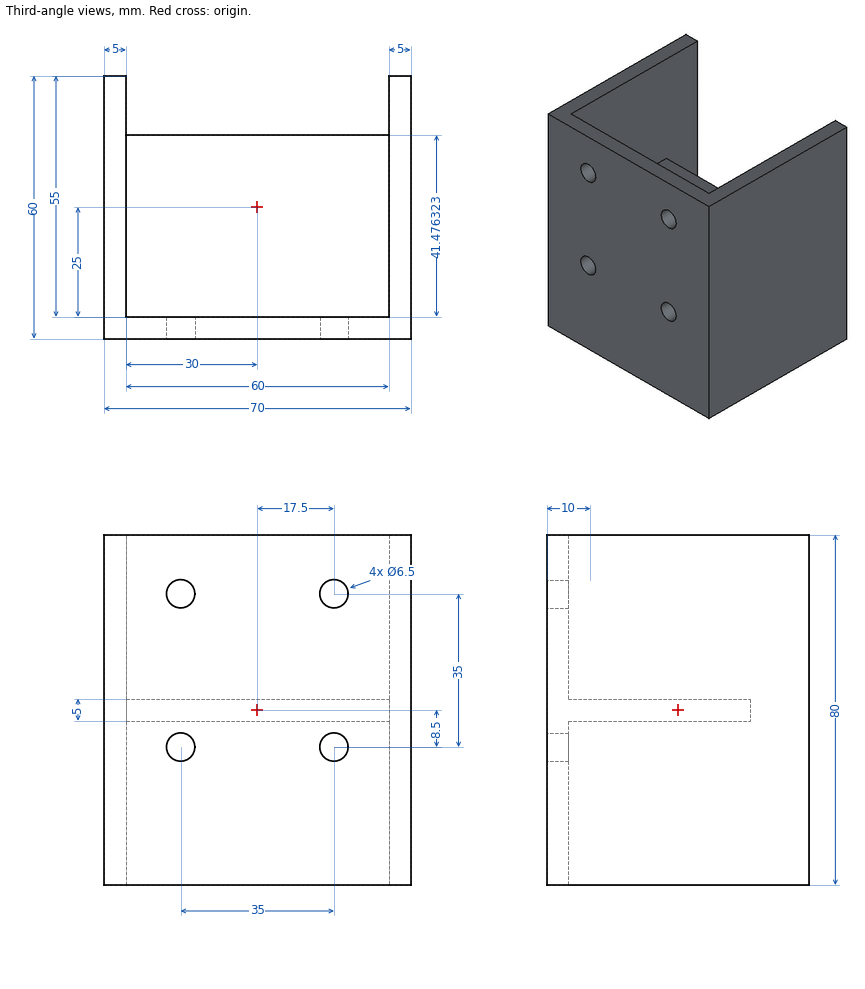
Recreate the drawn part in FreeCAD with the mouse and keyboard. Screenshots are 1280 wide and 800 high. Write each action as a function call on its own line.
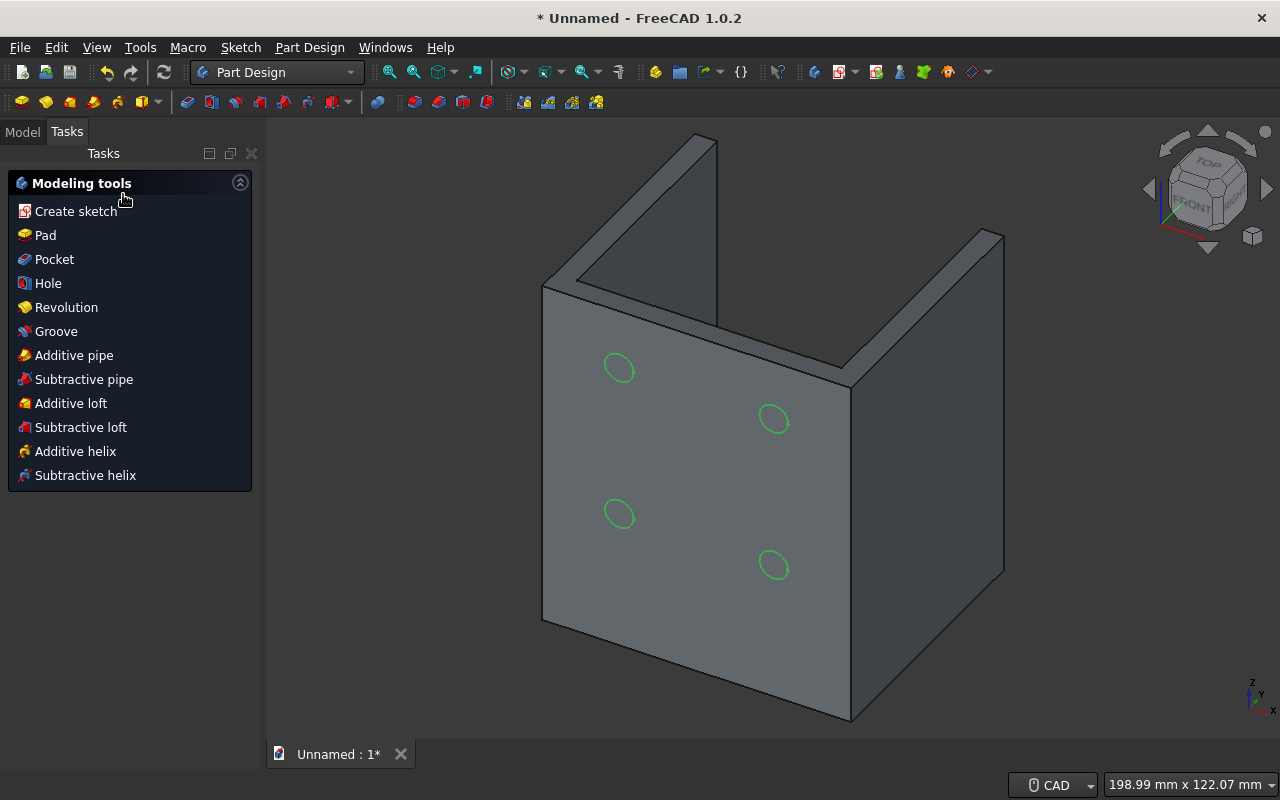
click(188, 102)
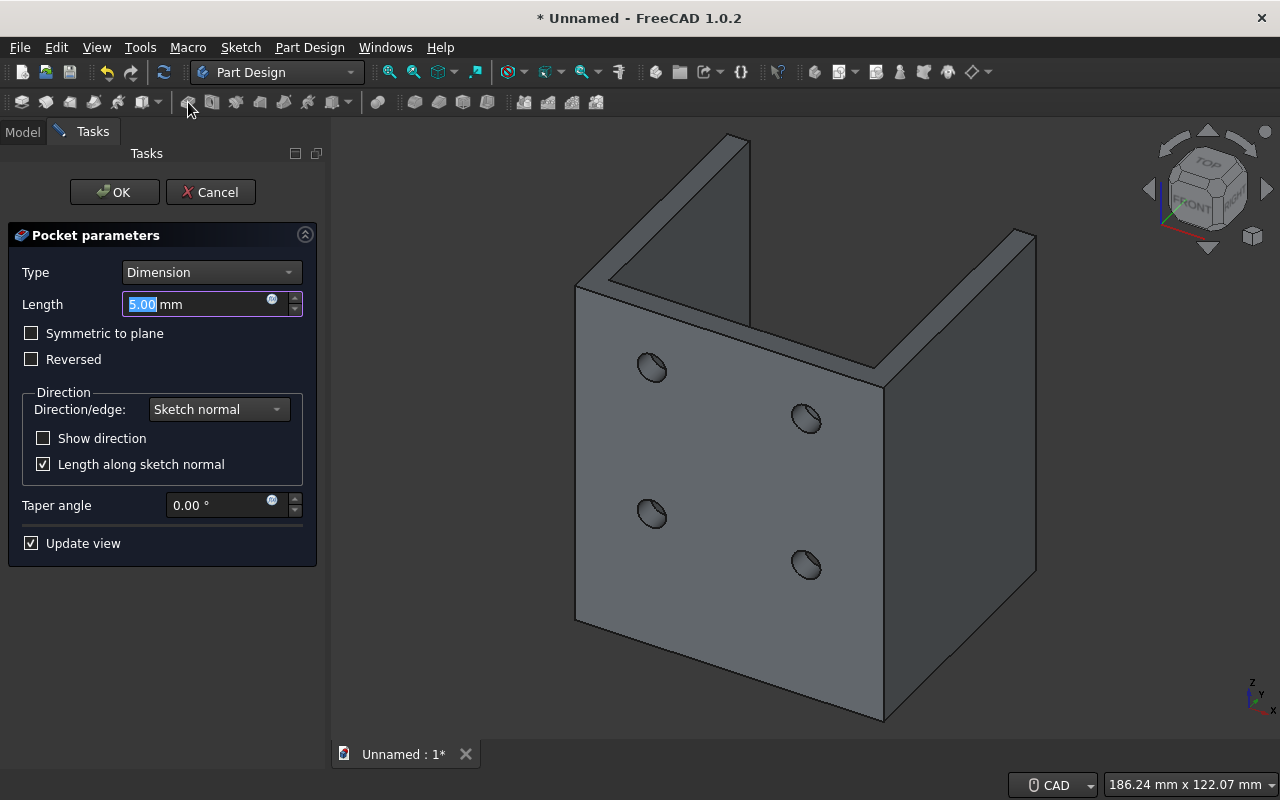
text(10)
key(Tab)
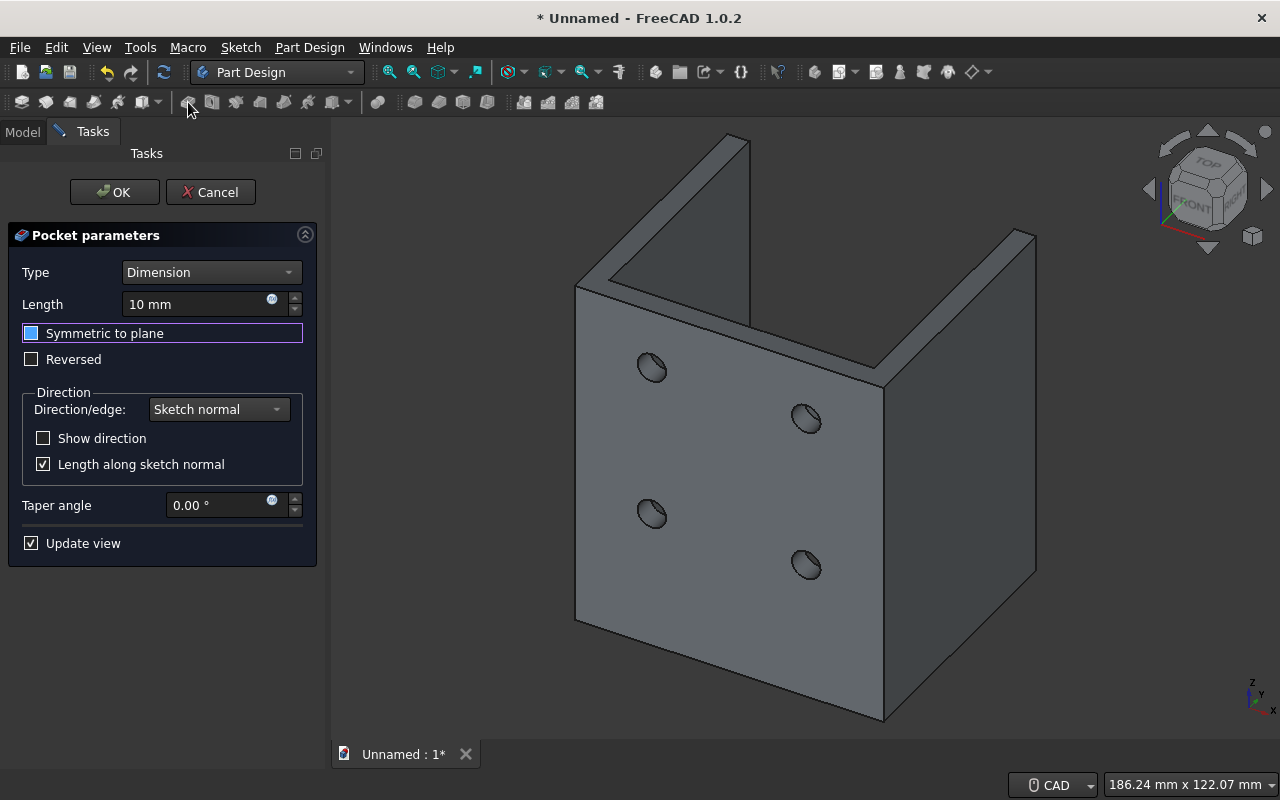
click(115, 192)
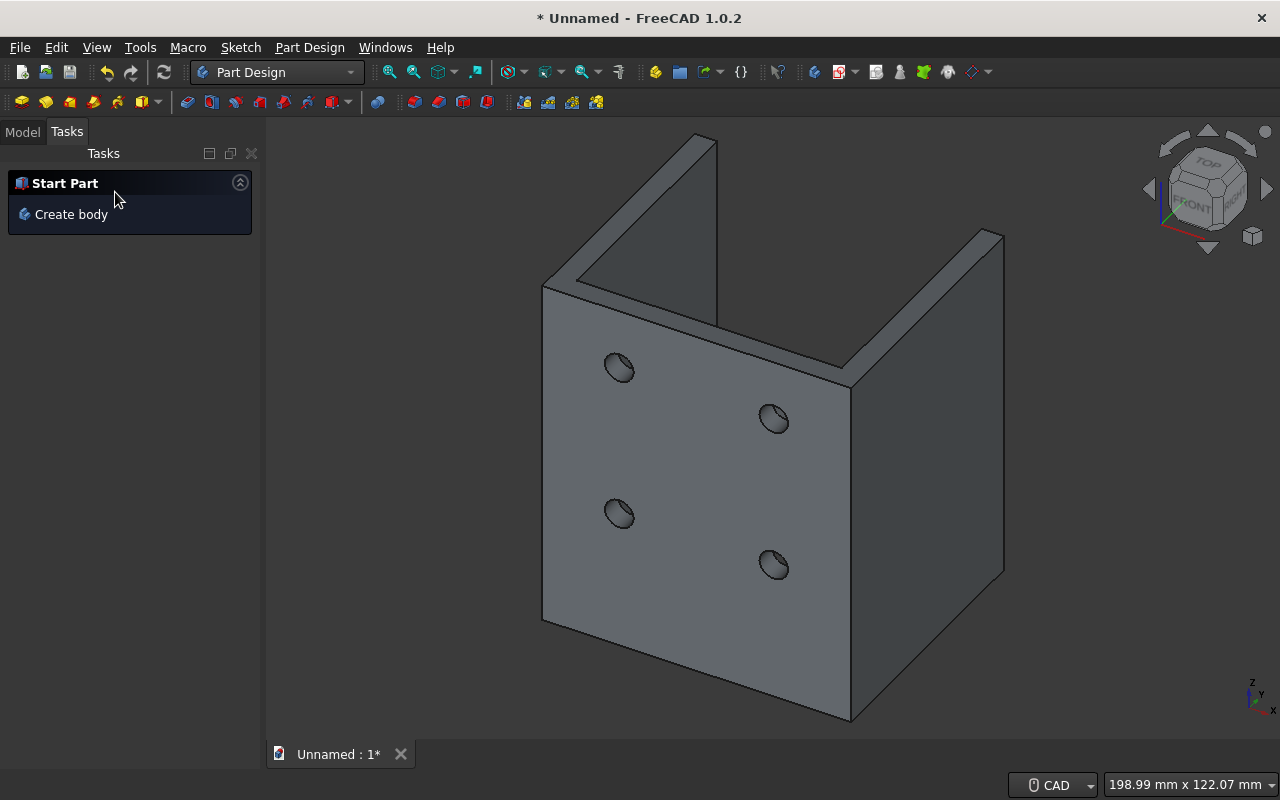
key(0)